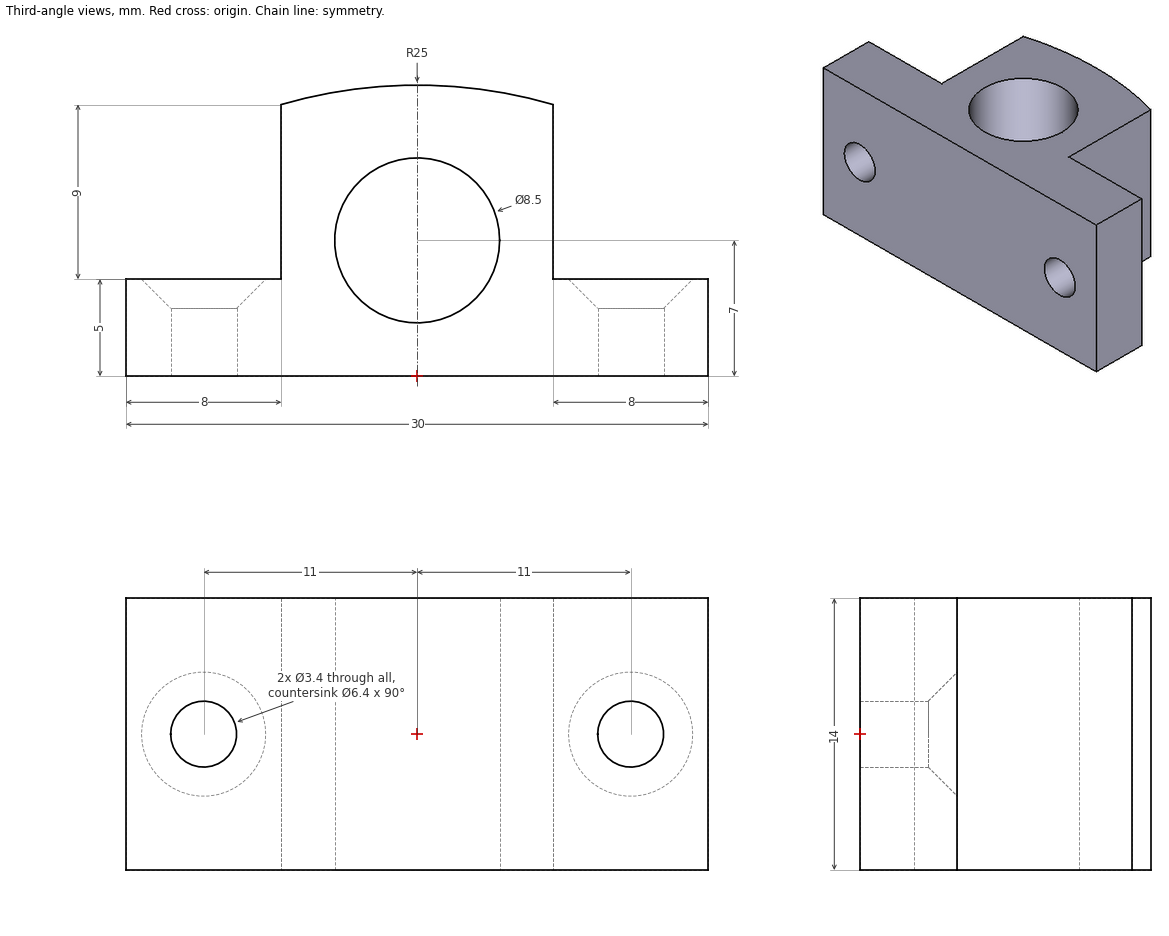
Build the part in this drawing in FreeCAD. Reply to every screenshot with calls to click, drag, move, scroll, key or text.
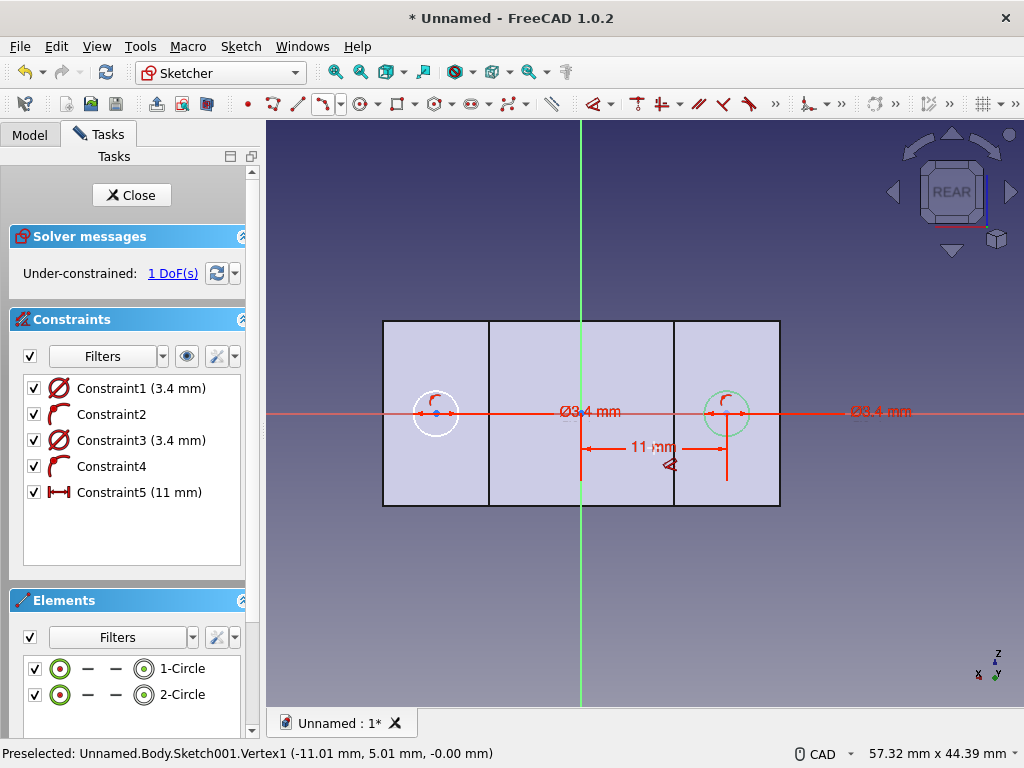
click(436, 414)
click(509, 448)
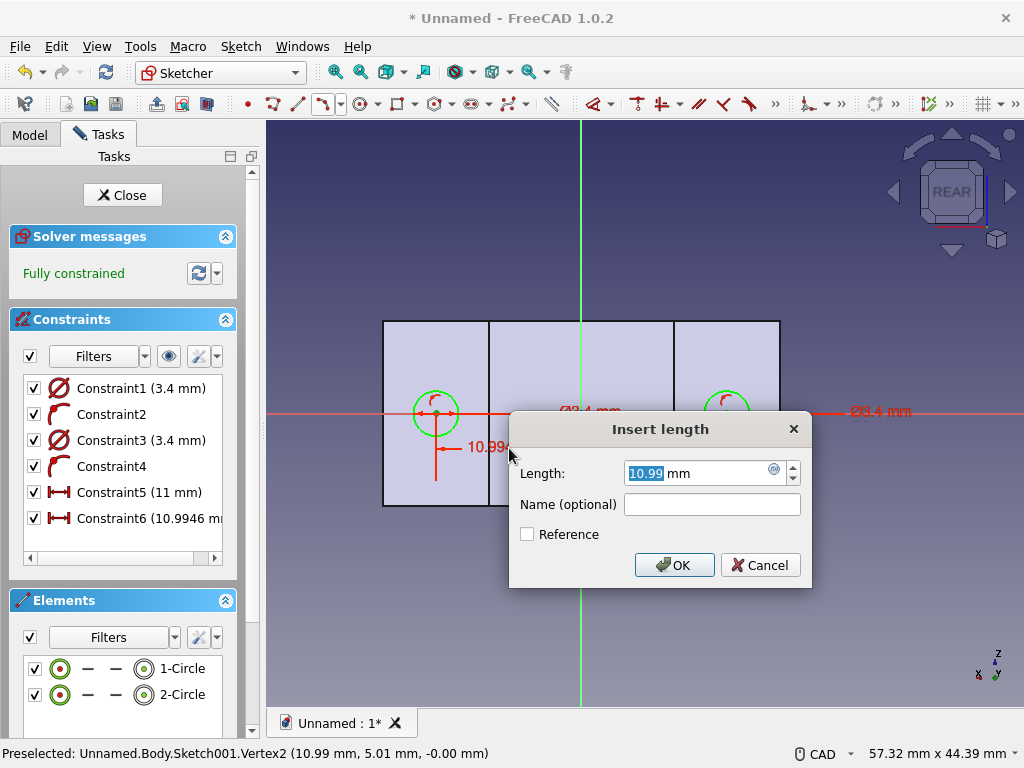
text(11)
key(Return)
key(Escape)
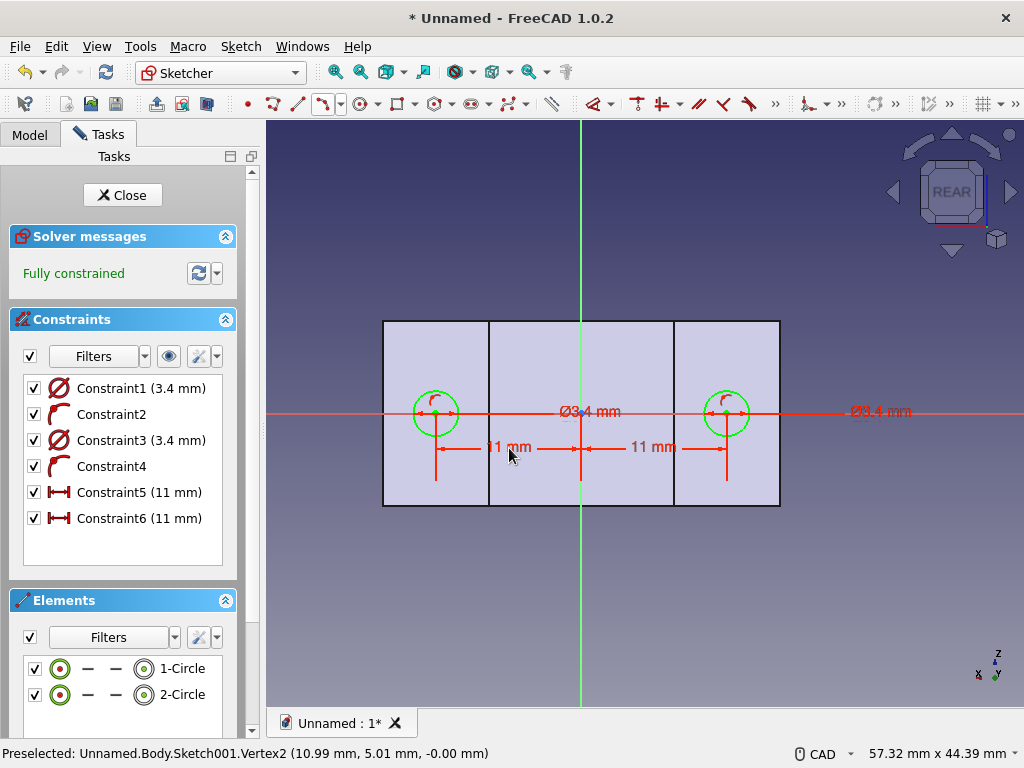
click(123, 195)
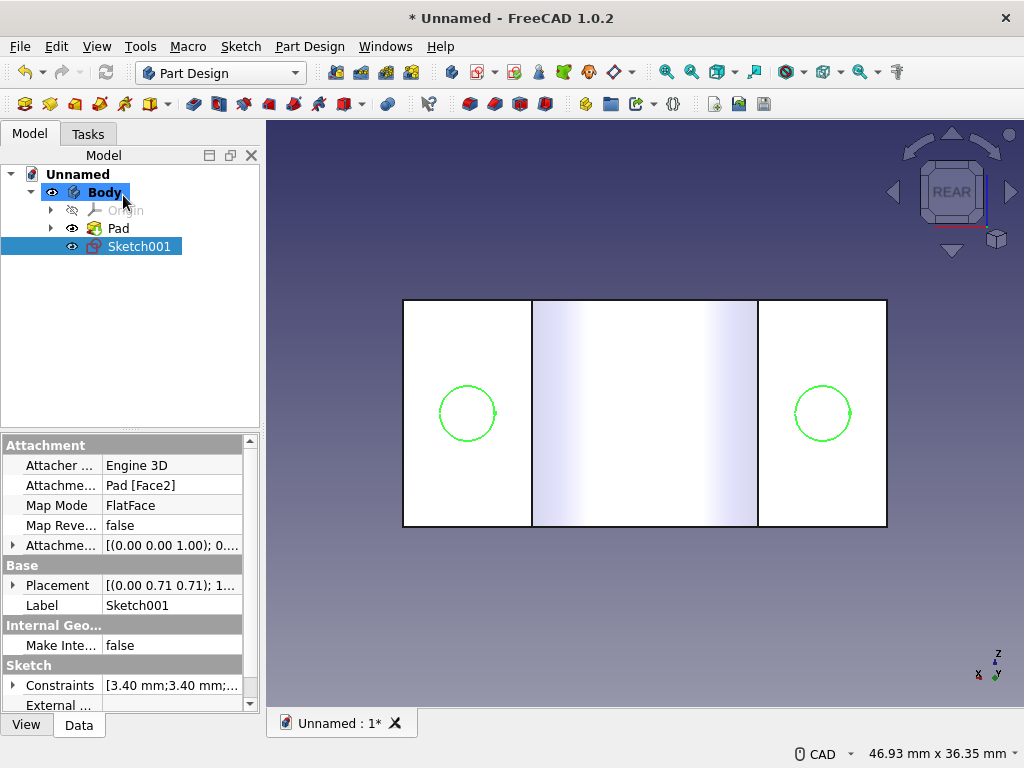
click(219, 104)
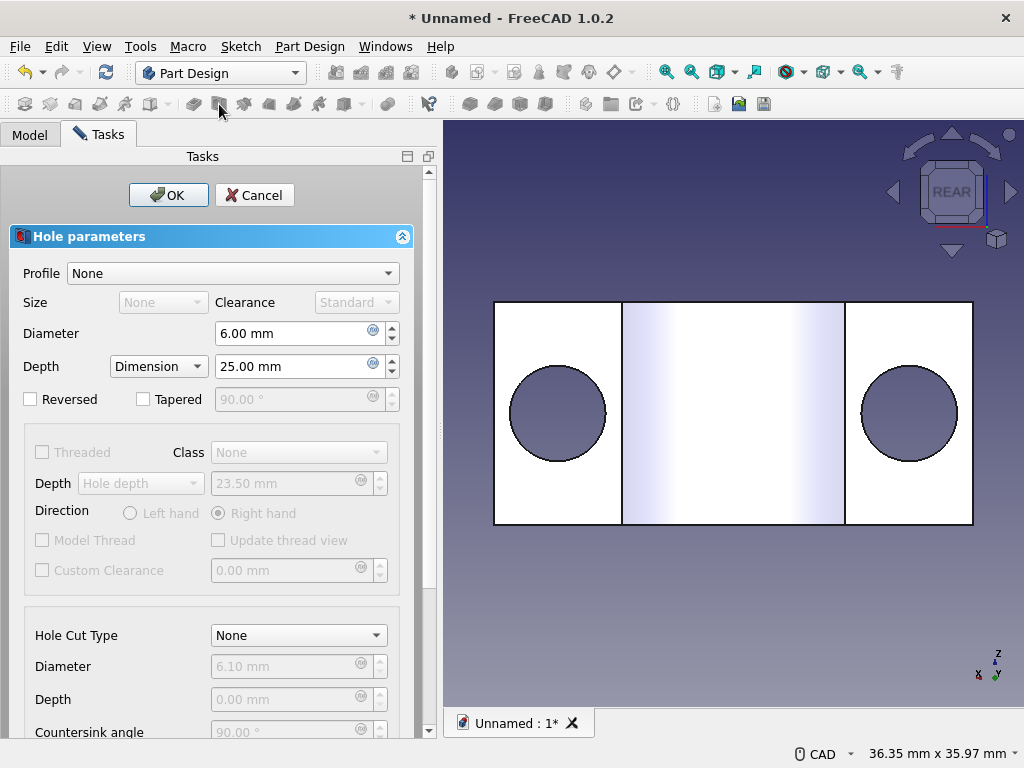
triple_click(300, 334)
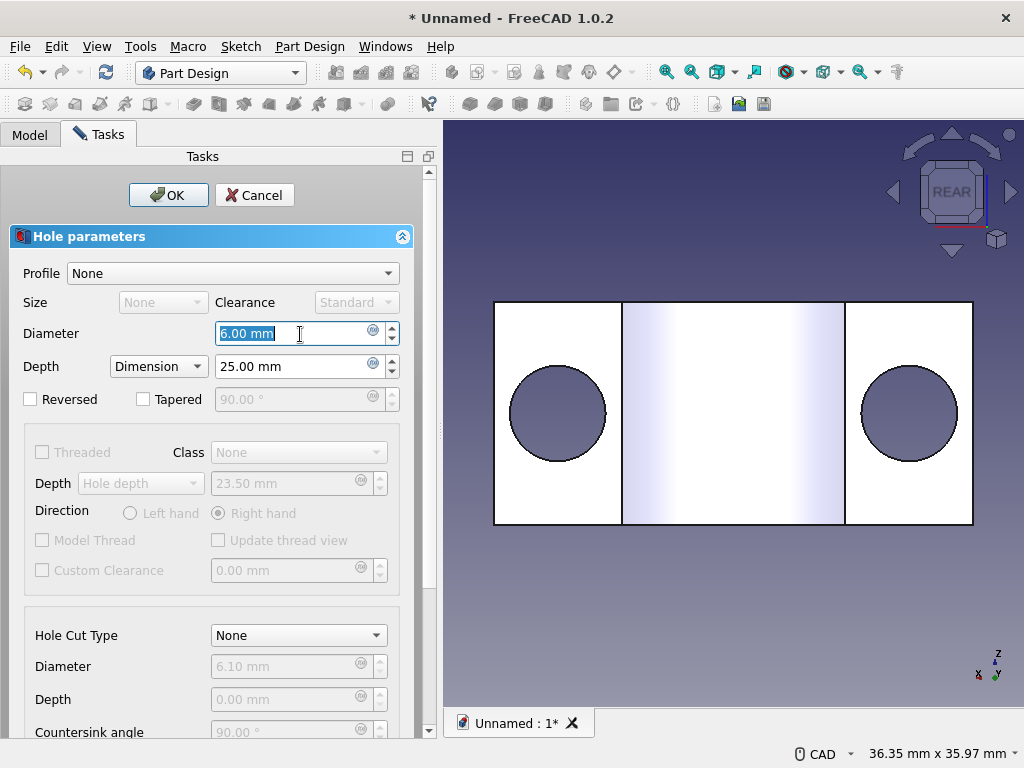
text(3.4)
key(Tab)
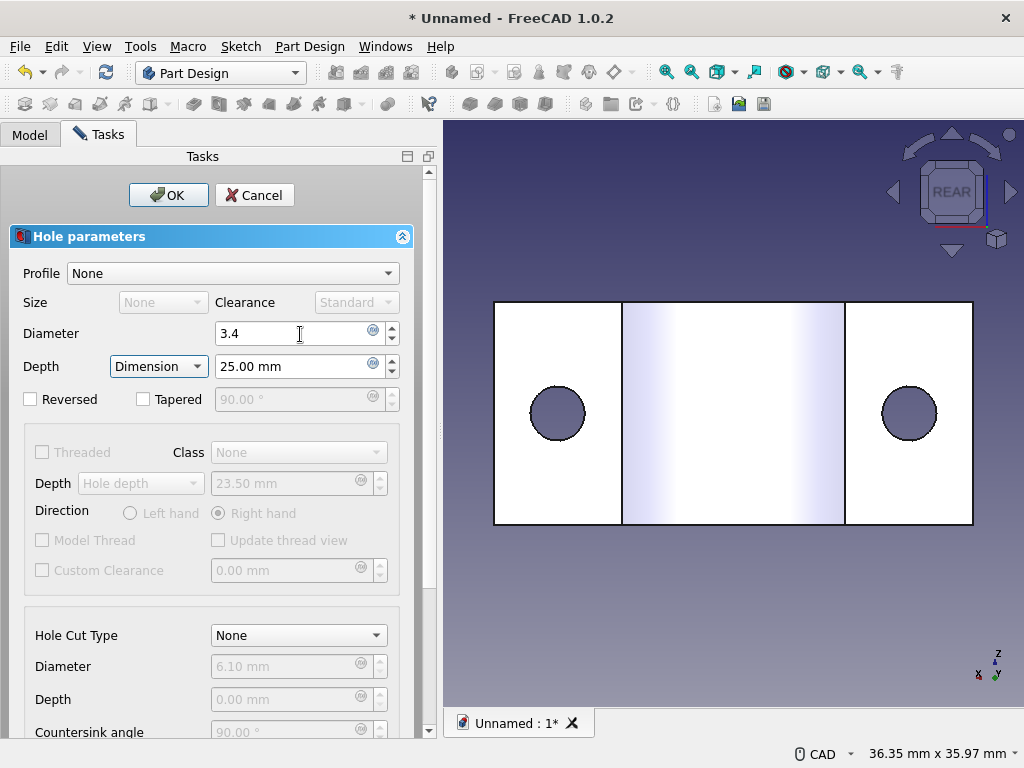
click(160, 366)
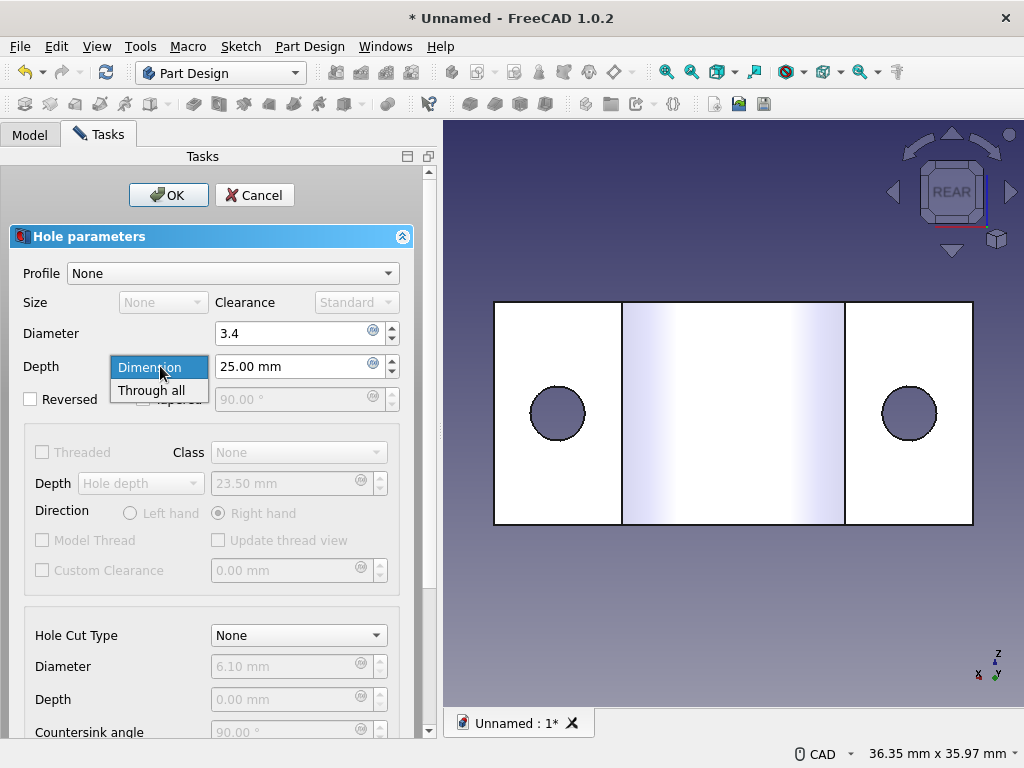
click(158, 390)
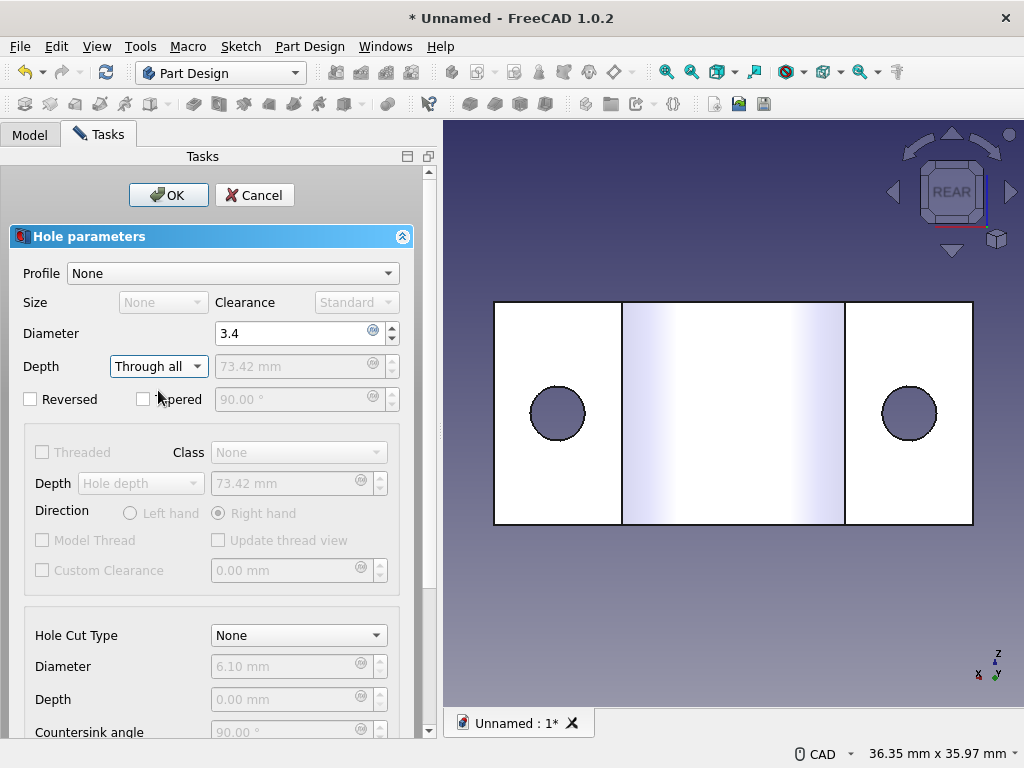
click(300, 636)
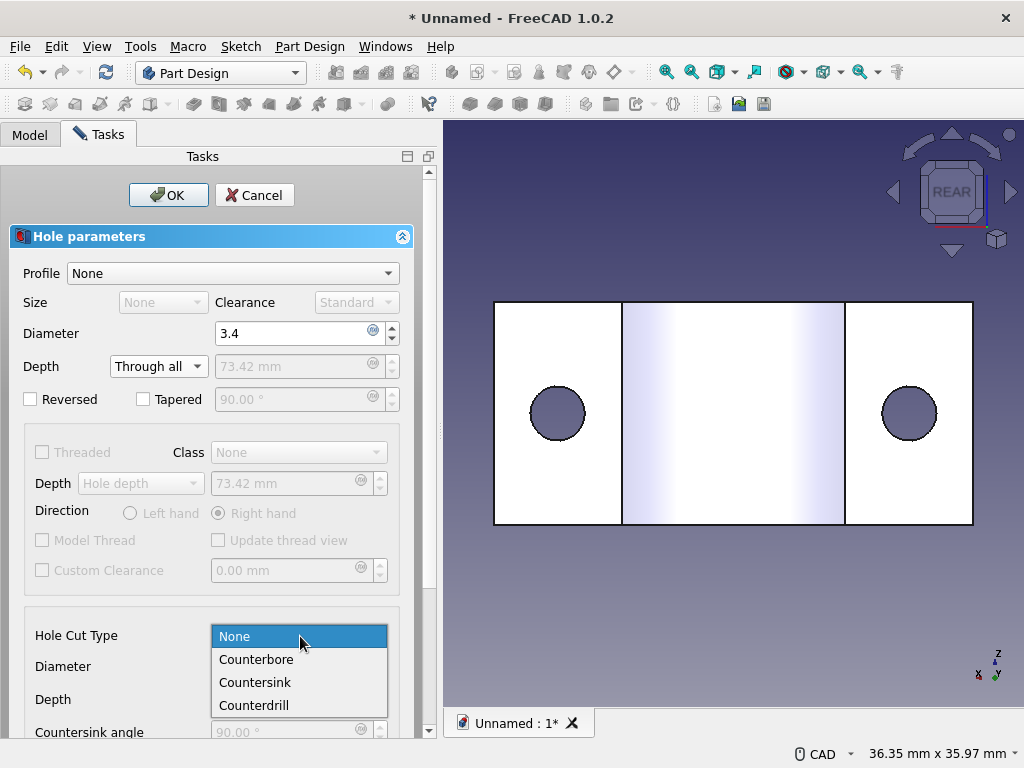
click(298, 682)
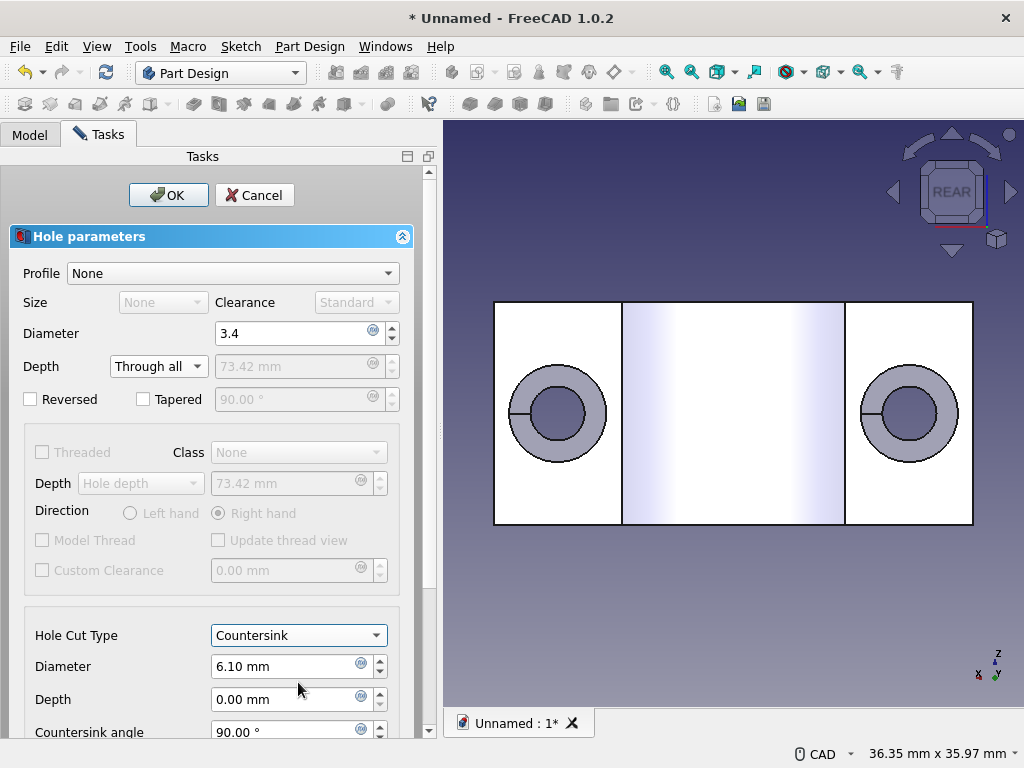
triple_click(292, 666)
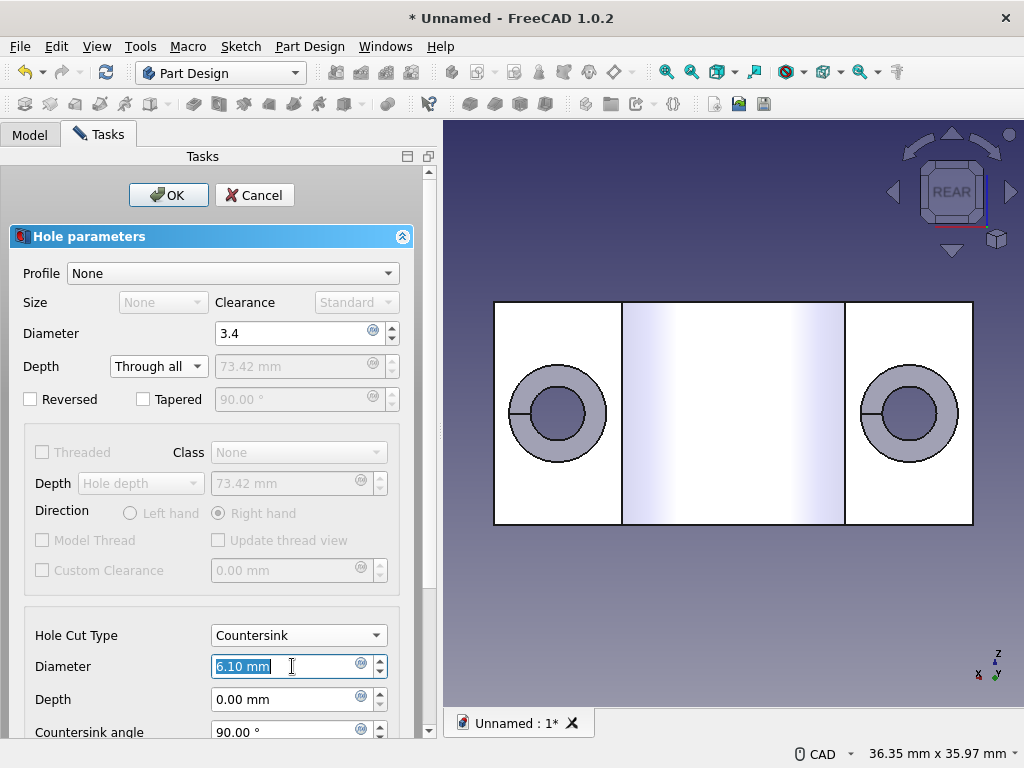
text(6.4)
key(Tab)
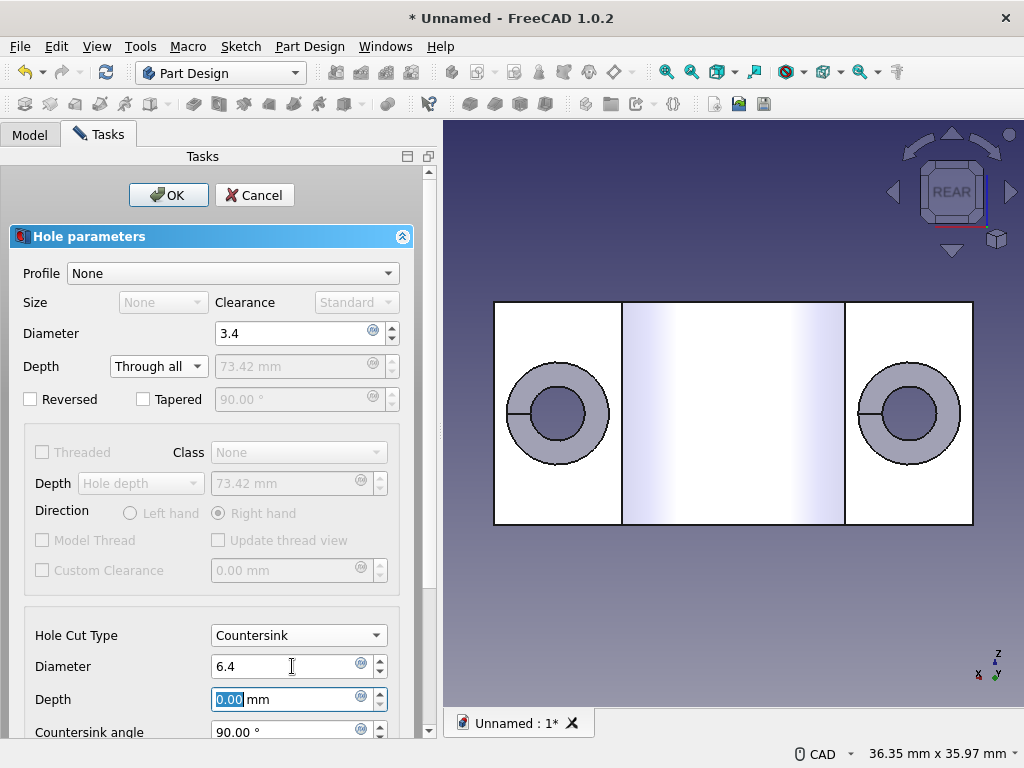
click(169, 195)